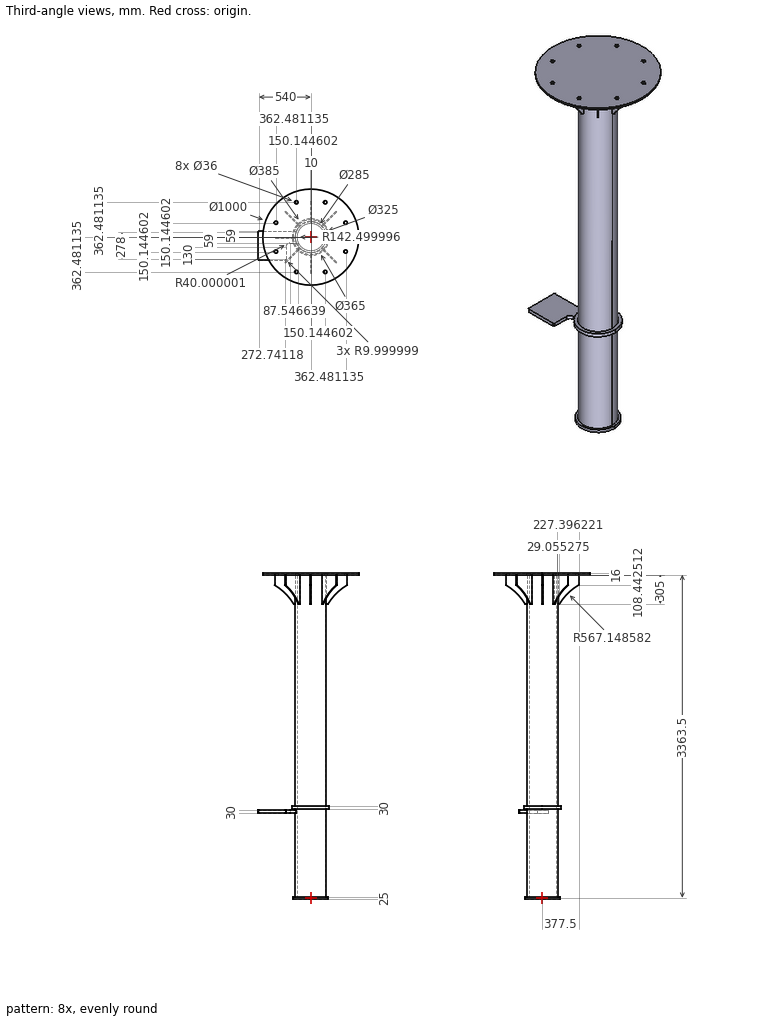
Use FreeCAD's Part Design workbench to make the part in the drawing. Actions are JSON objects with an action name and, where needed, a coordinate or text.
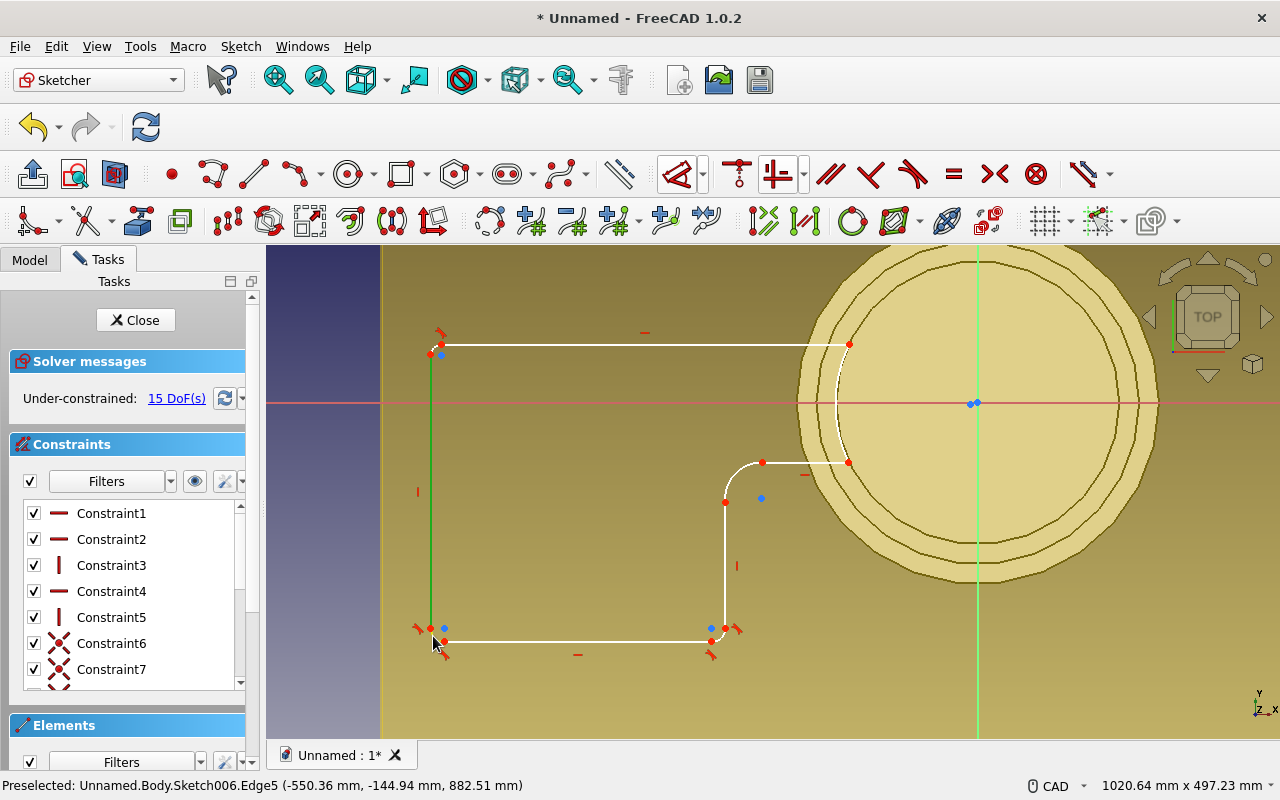
{"action": "scroll", "coordinate": [437, 346], "scroll_direction": "up", "scroll_amount": 6}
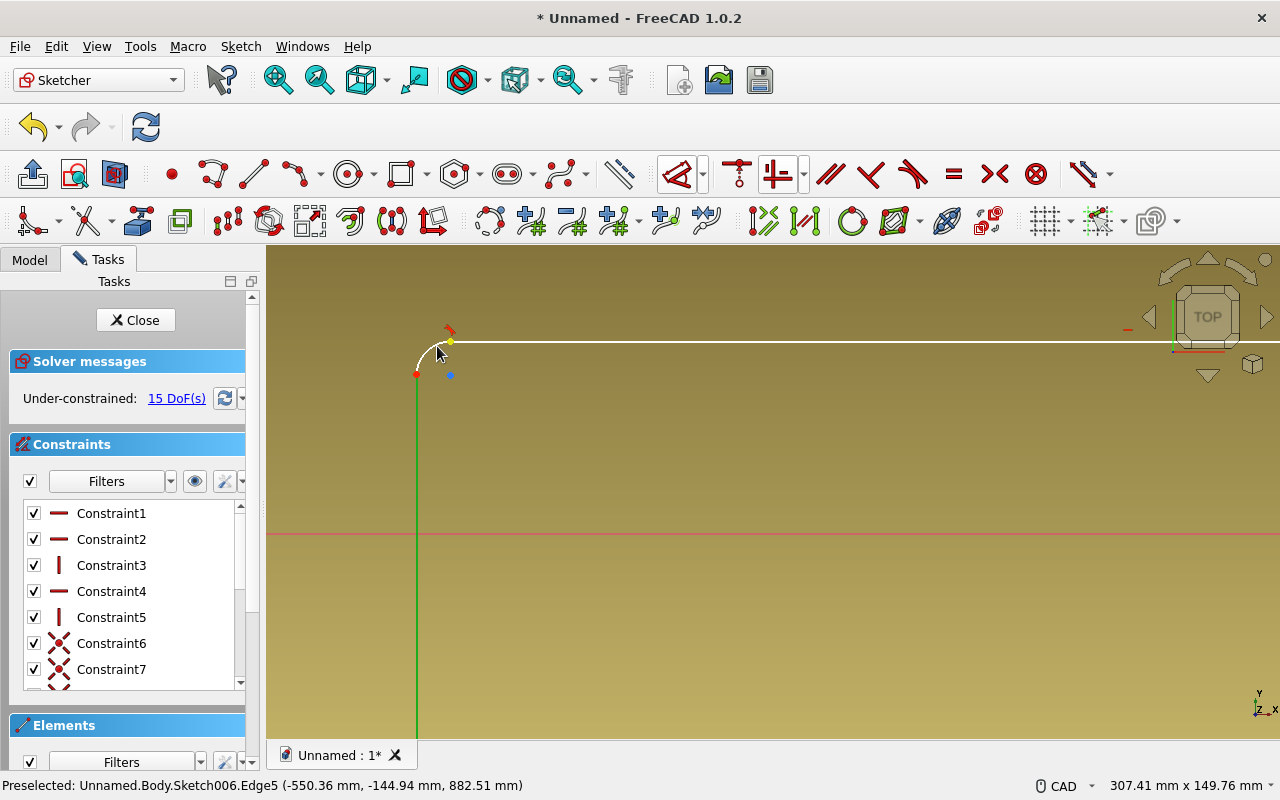
{"action": "left_click", "coordinate": [436, 345]}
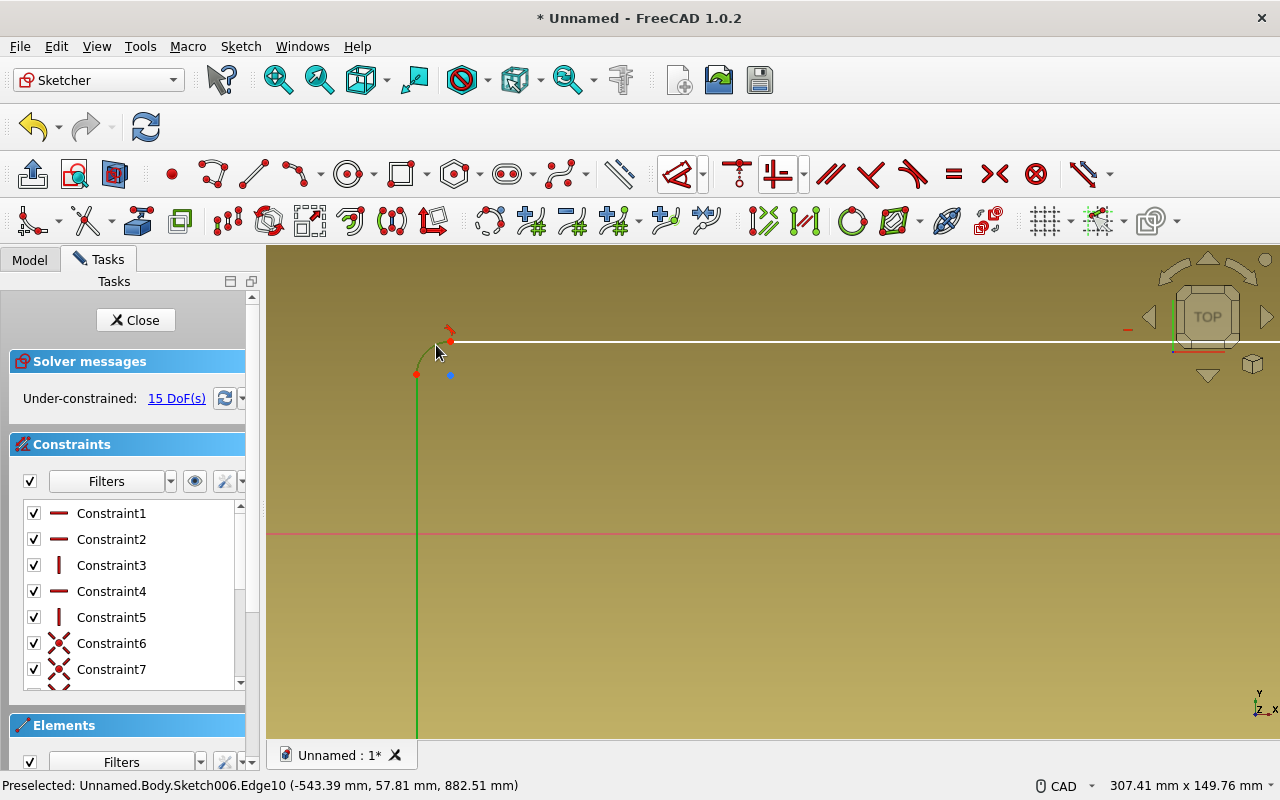
{"action": "key", "text": "t"}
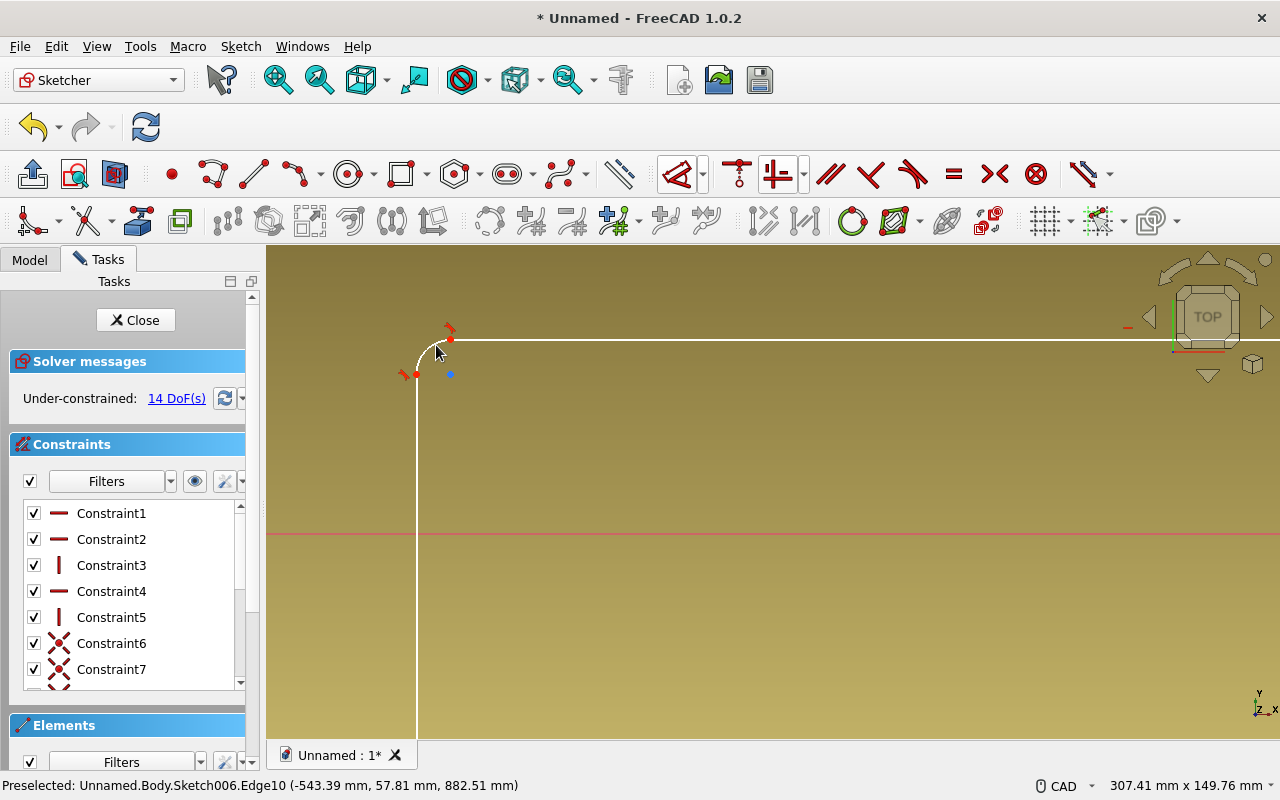
{"action": "scroll", "coordinate": [437, 346], "scroll_direction": "down", "scroll_amount": 6}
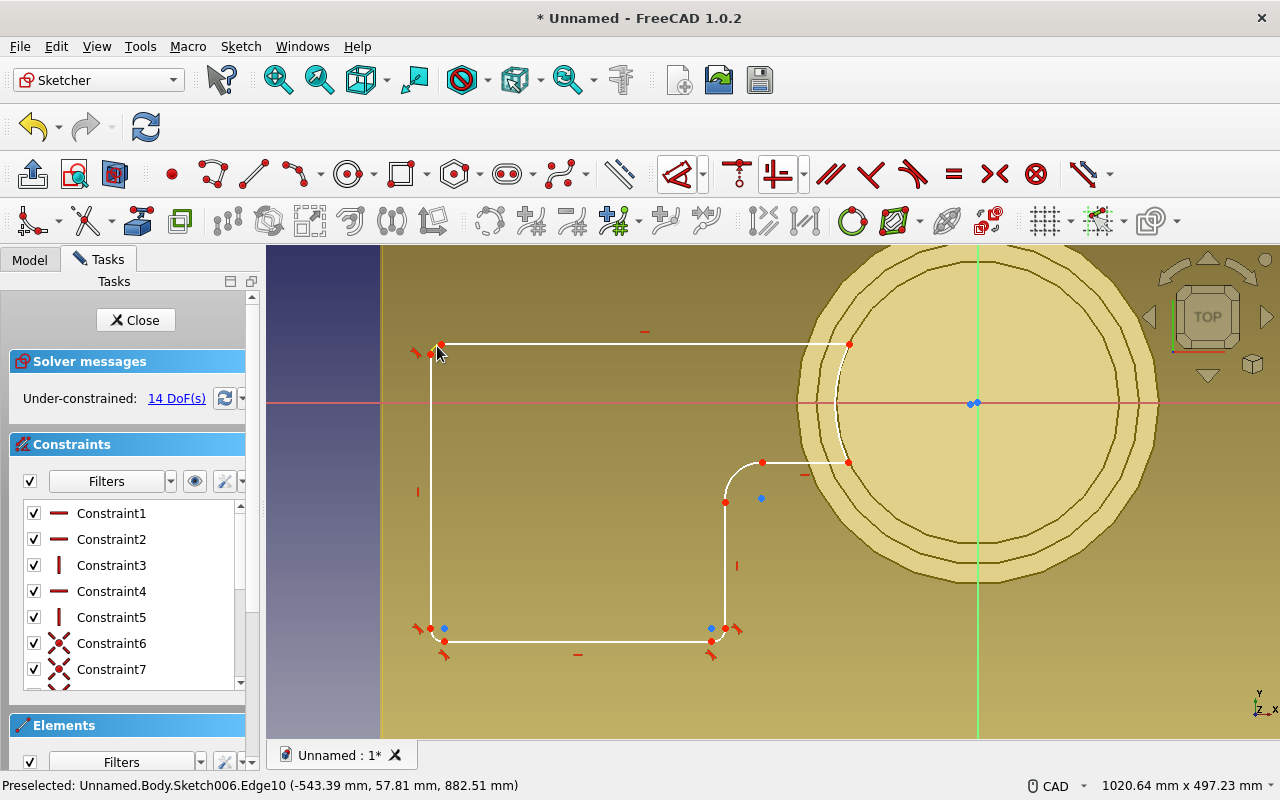
{"action": "scroll", "coordinate": [974, 403], "scroll_direction": "up", "scroll_amount": 7}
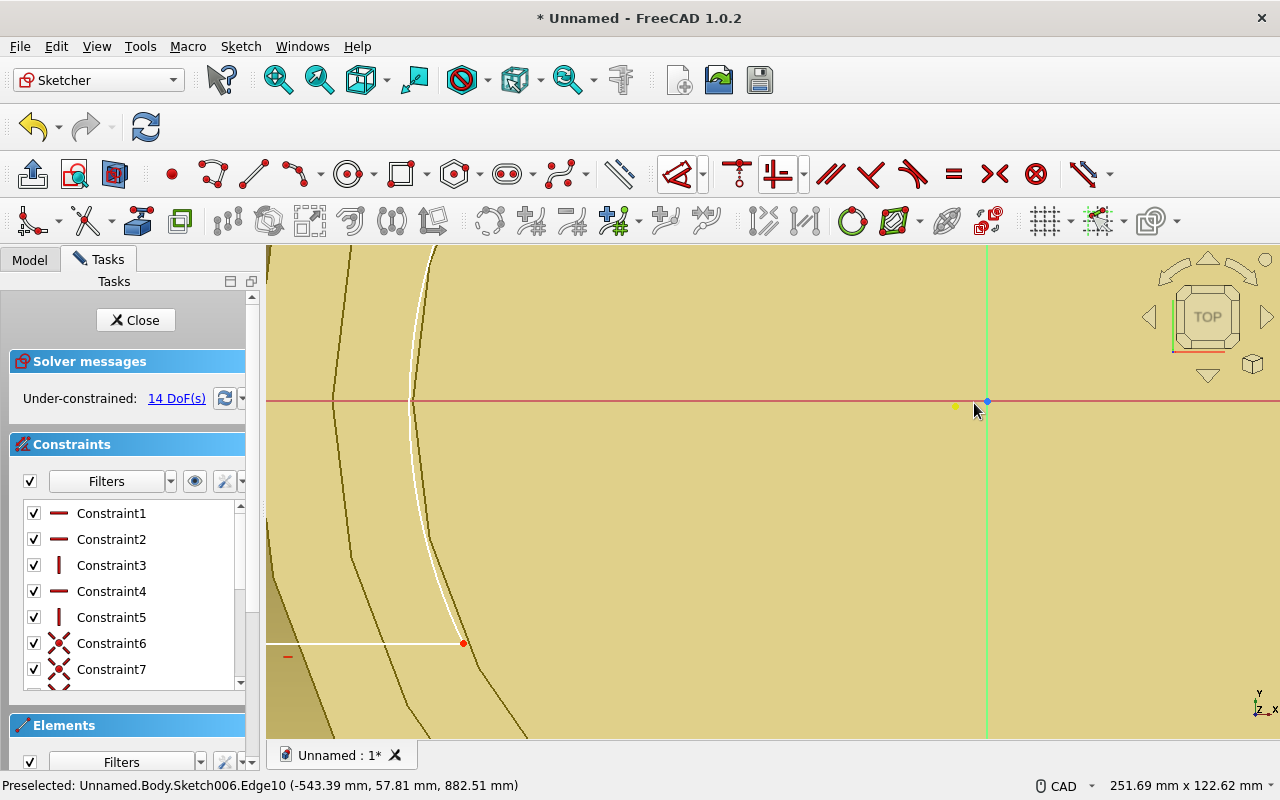
{"action": "left_click_drag", "start_coordinate": [946, 391], "coordinate": [997, 417]}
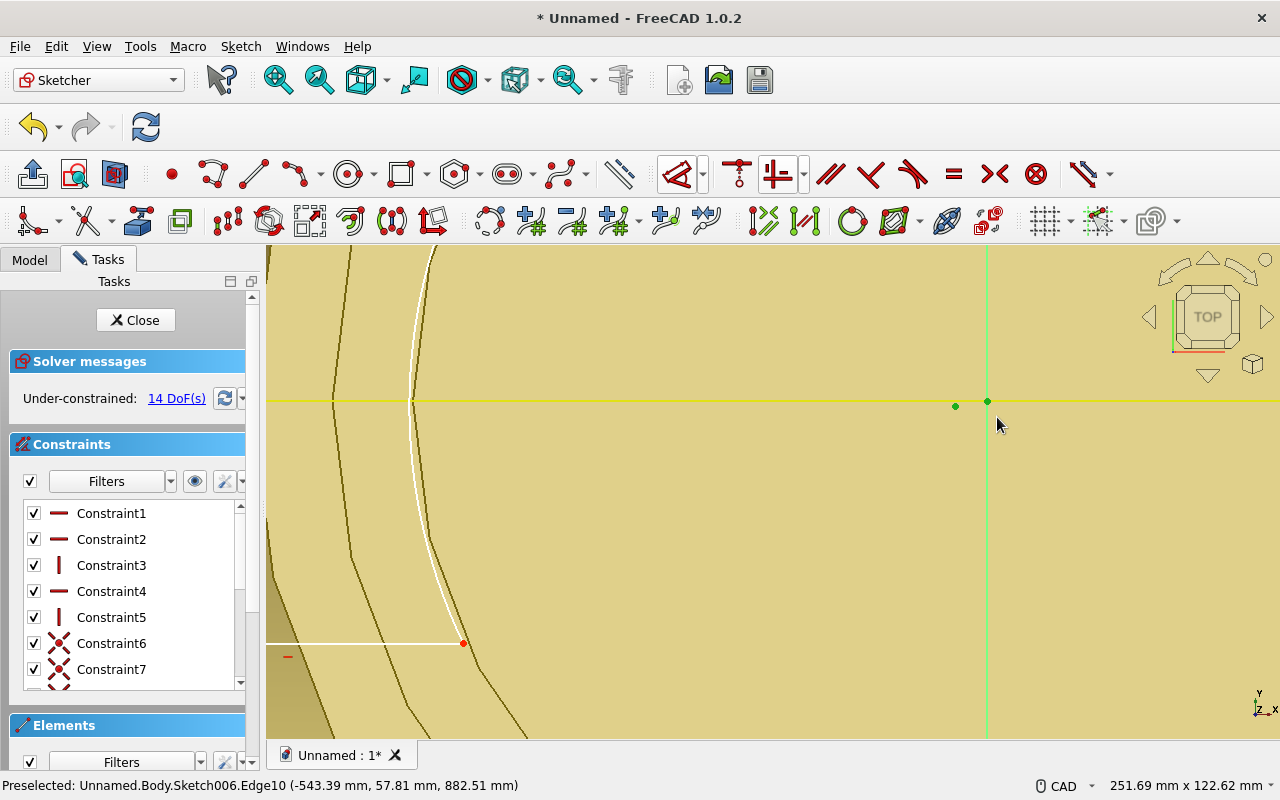
{"action": "key", "text": "c"}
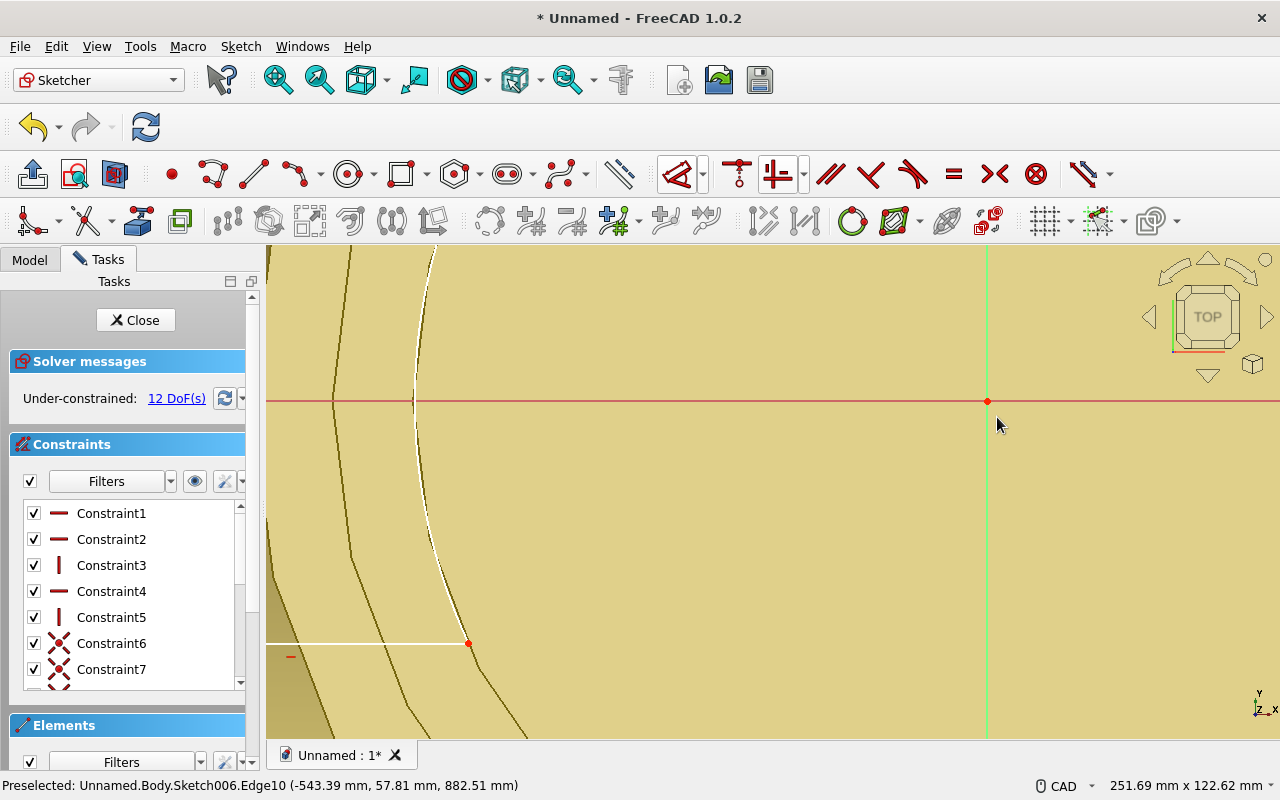
{"action": "scroll", "coordinate": [975, 403], "scroll_direction": "down", "scroll_amount": 7}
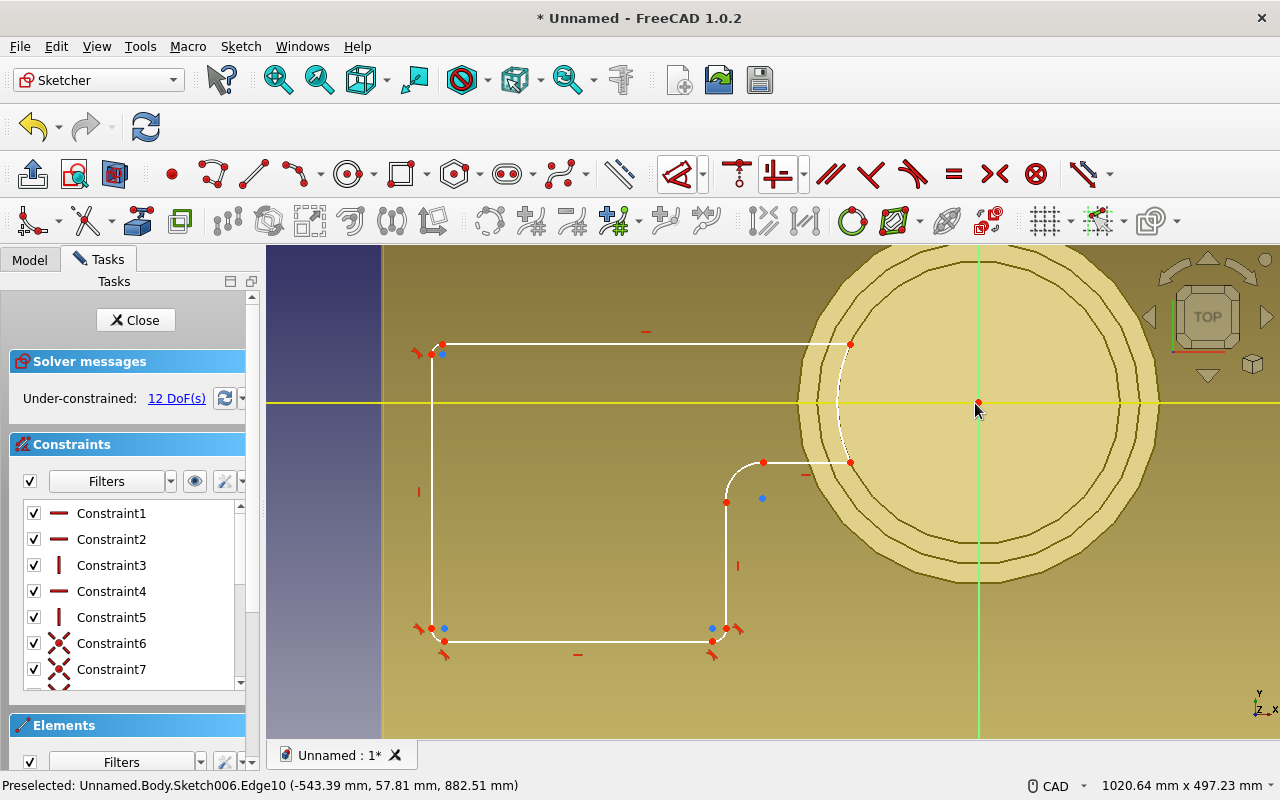
{"action": "scroll", "coordinate": [719, 640], "scroll_direction": "up", "scroll_amount": 4}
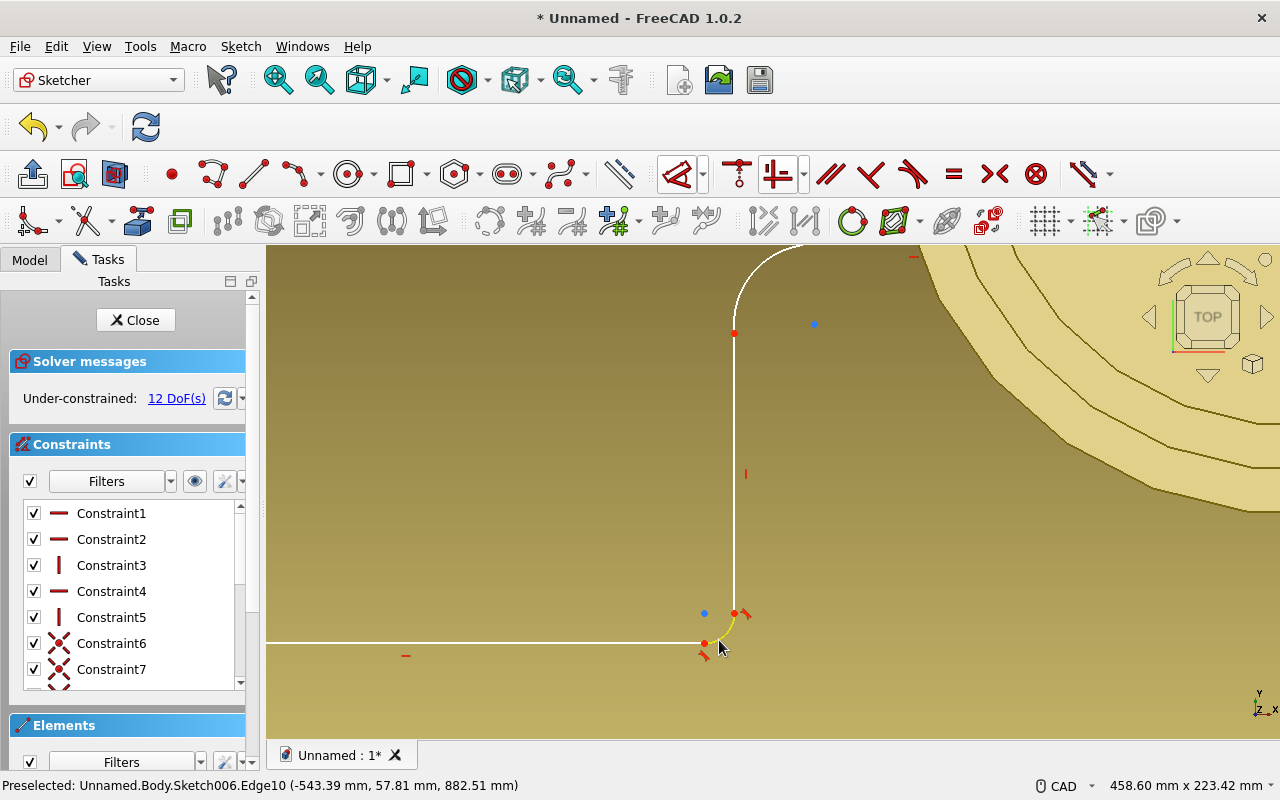
{"action": "left_click", "coordinate": [718, 640]}